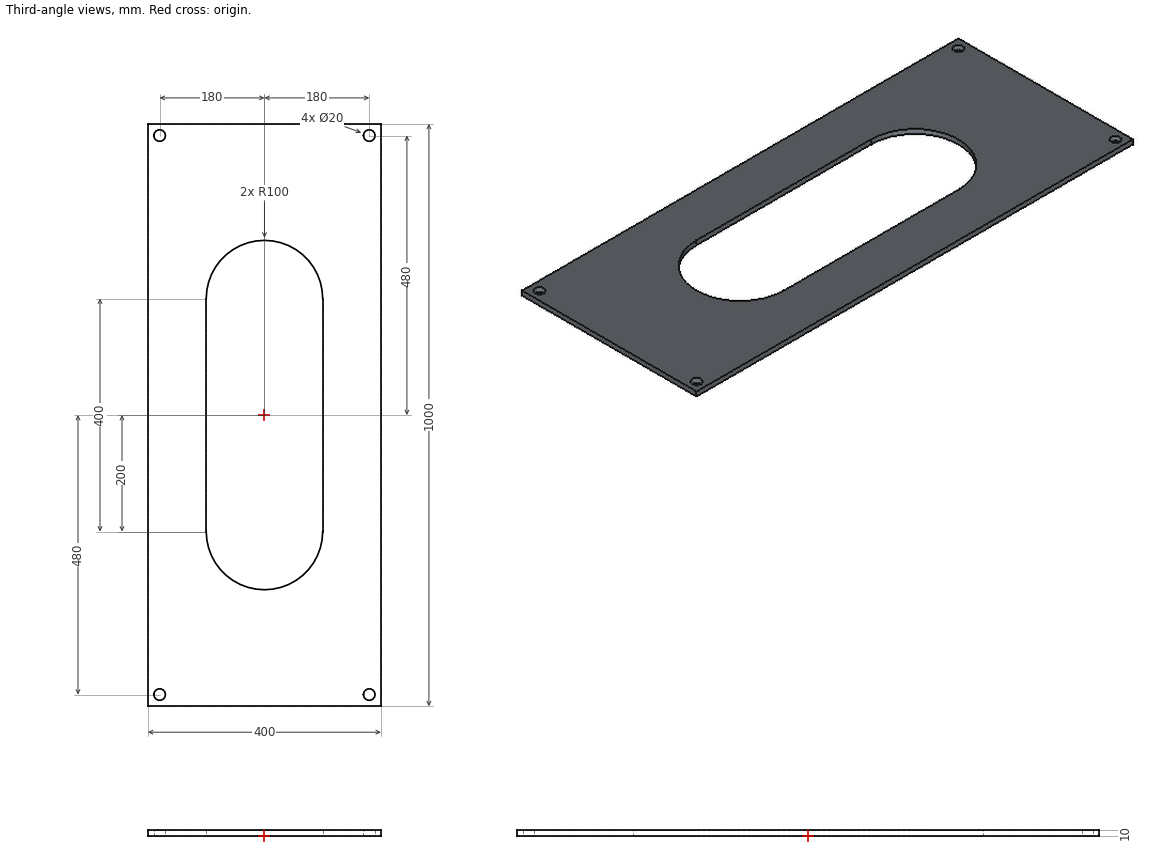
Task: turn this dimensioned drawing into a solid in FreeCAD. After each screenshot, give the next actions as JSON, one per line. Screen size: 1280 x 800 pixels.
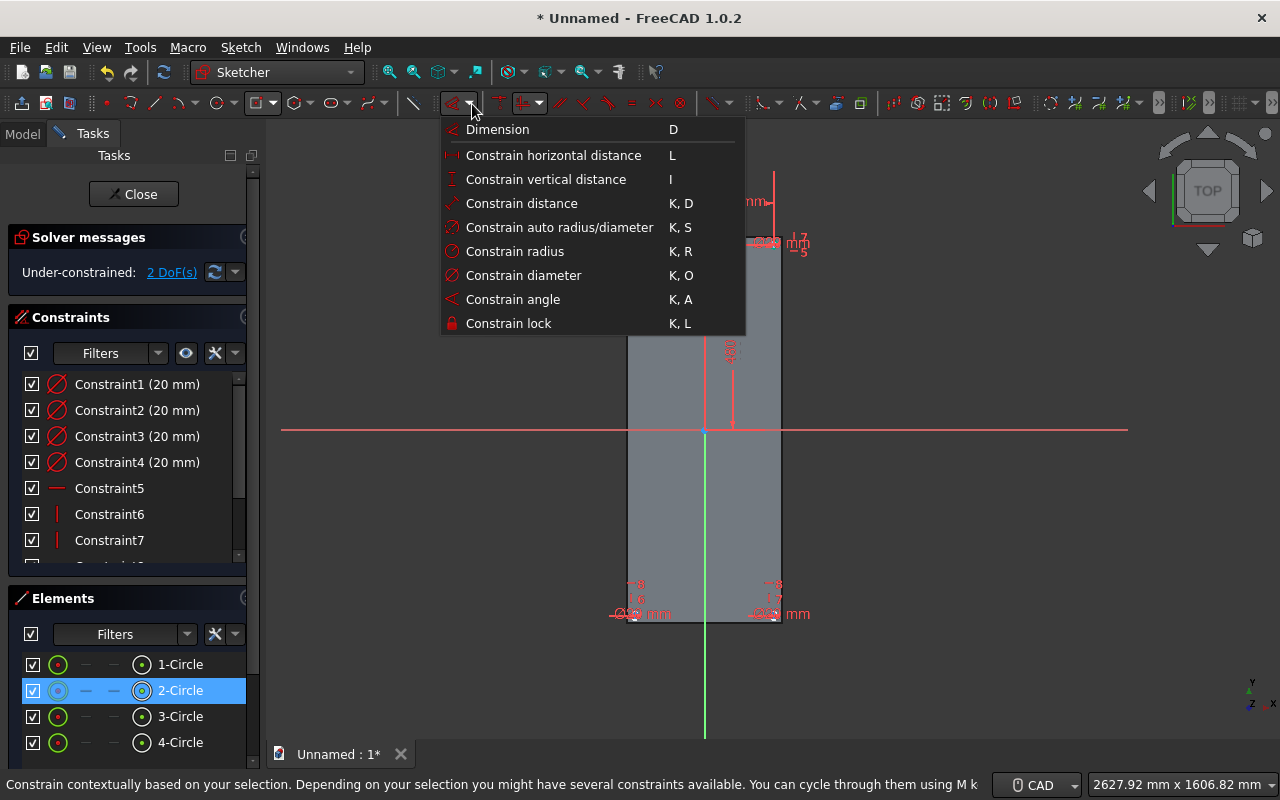
{"action": "left_click", "coordinate": [593, 155]}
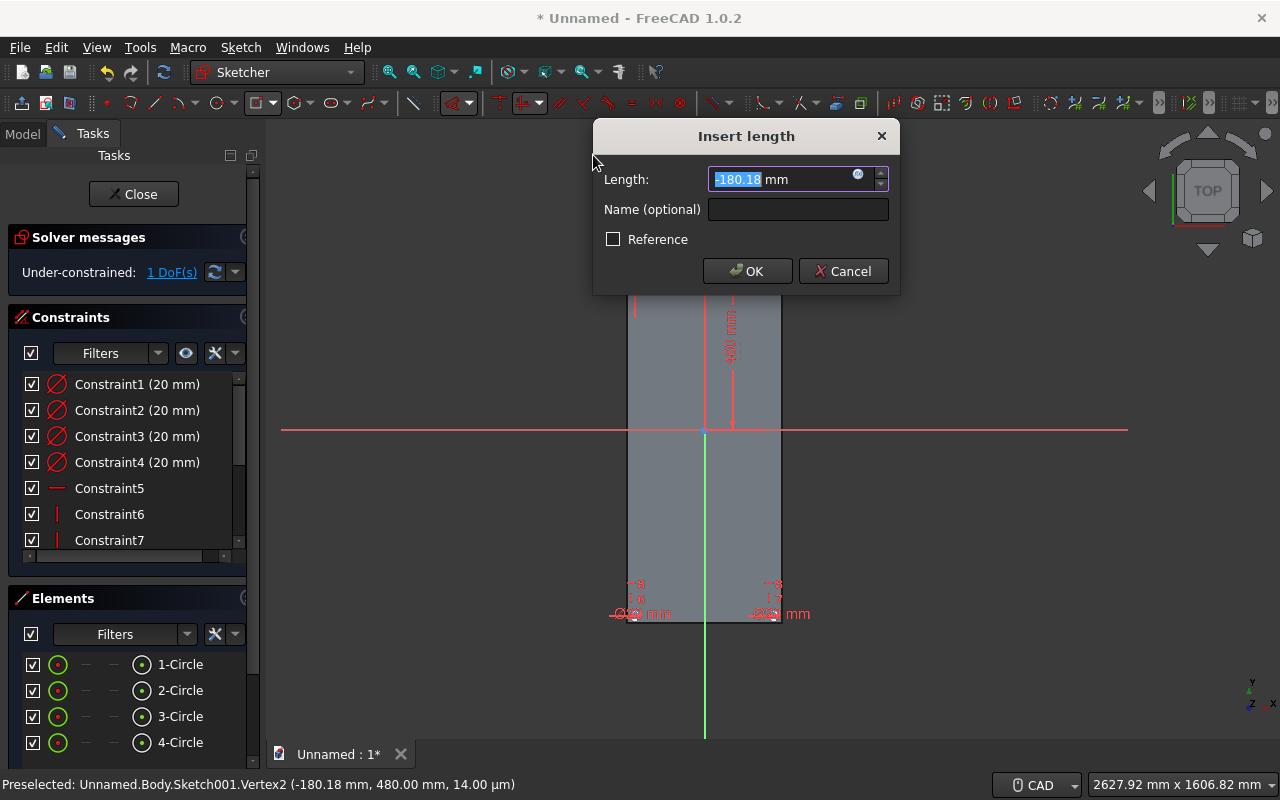
{"action": "type", "text": "-180"}
{"action": "key", "text": "Return"}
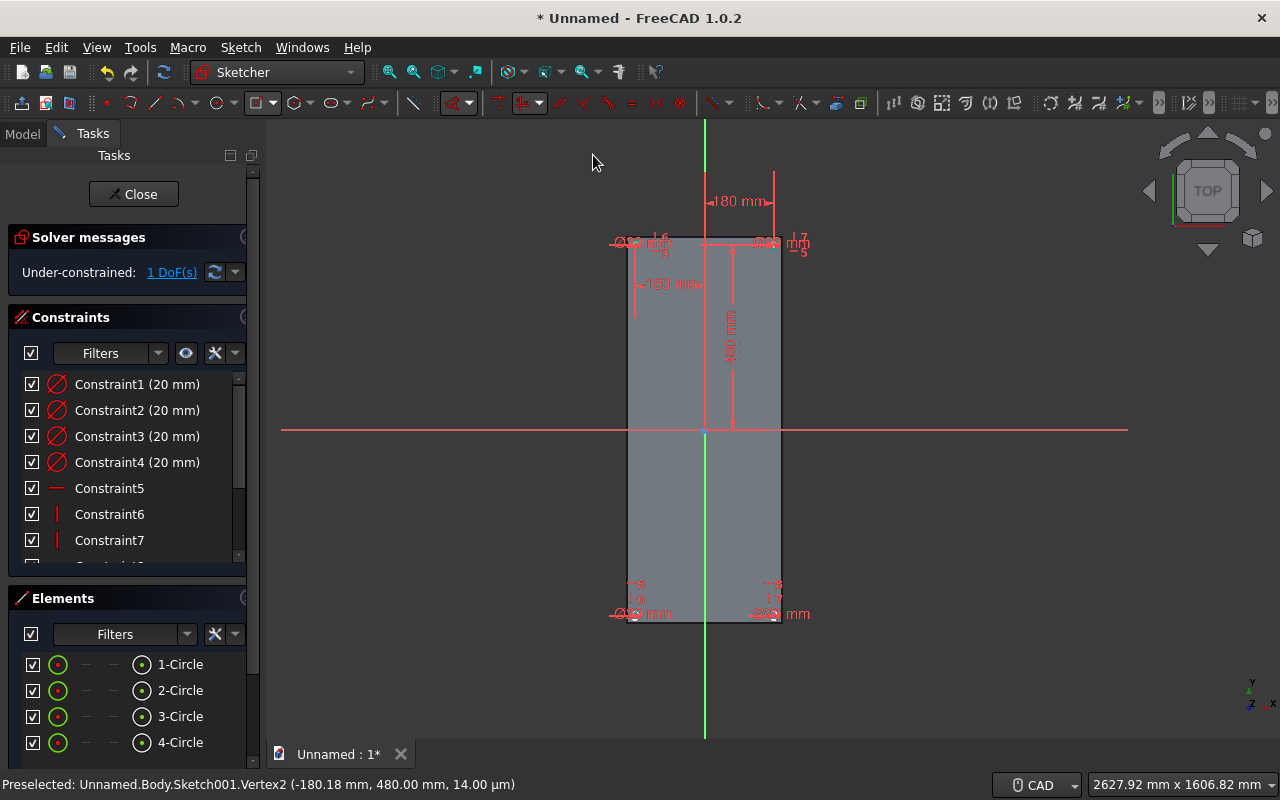
{"action": "left_click", "coordinate": [635, 616]}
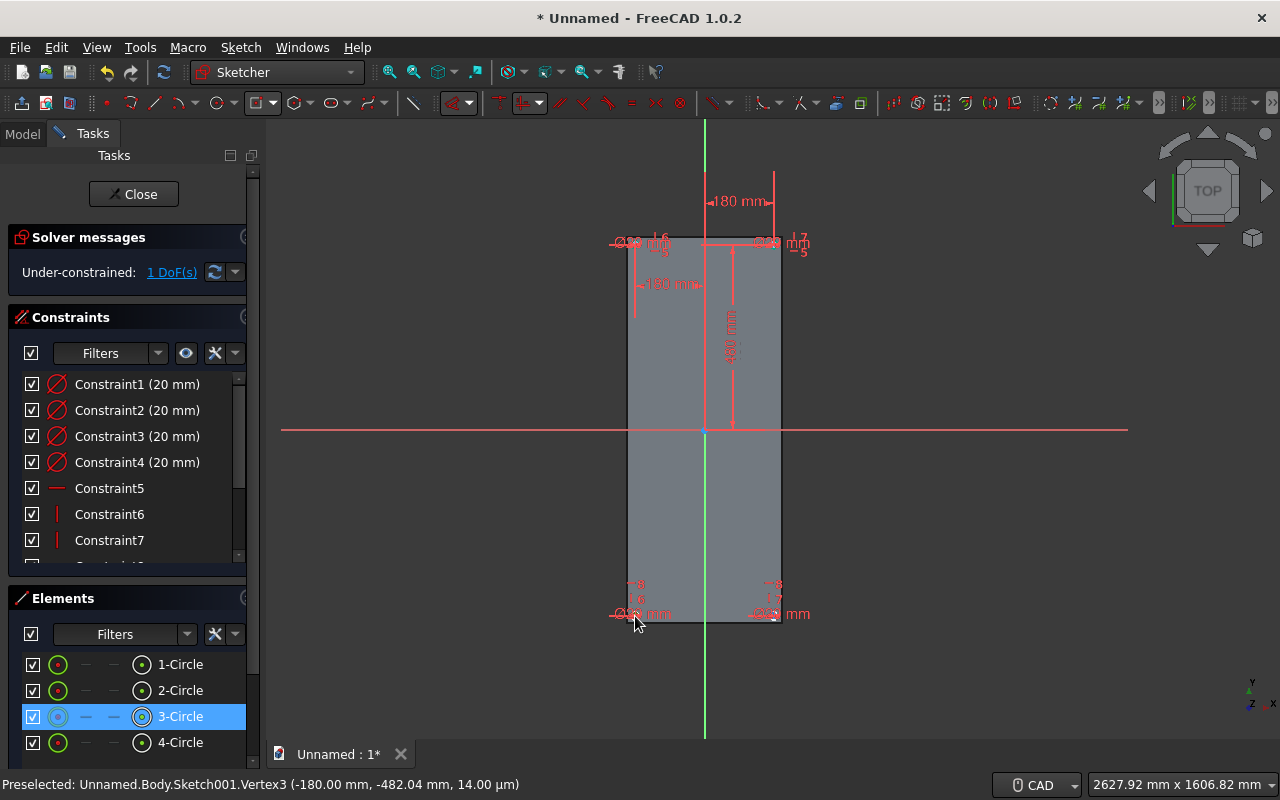
{"action": "left_click", "coordinate": [472, 104]}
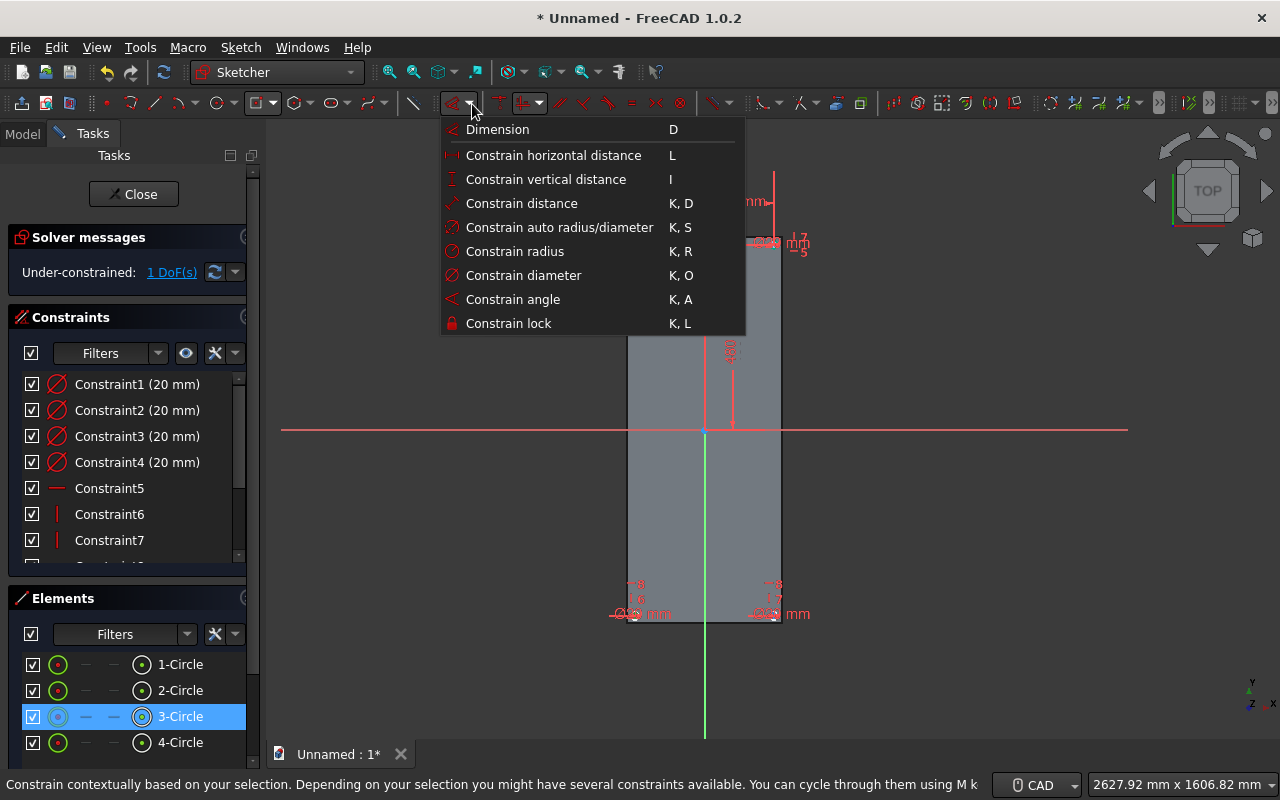
{"action": "left_click", "coordinate": [593, 179]}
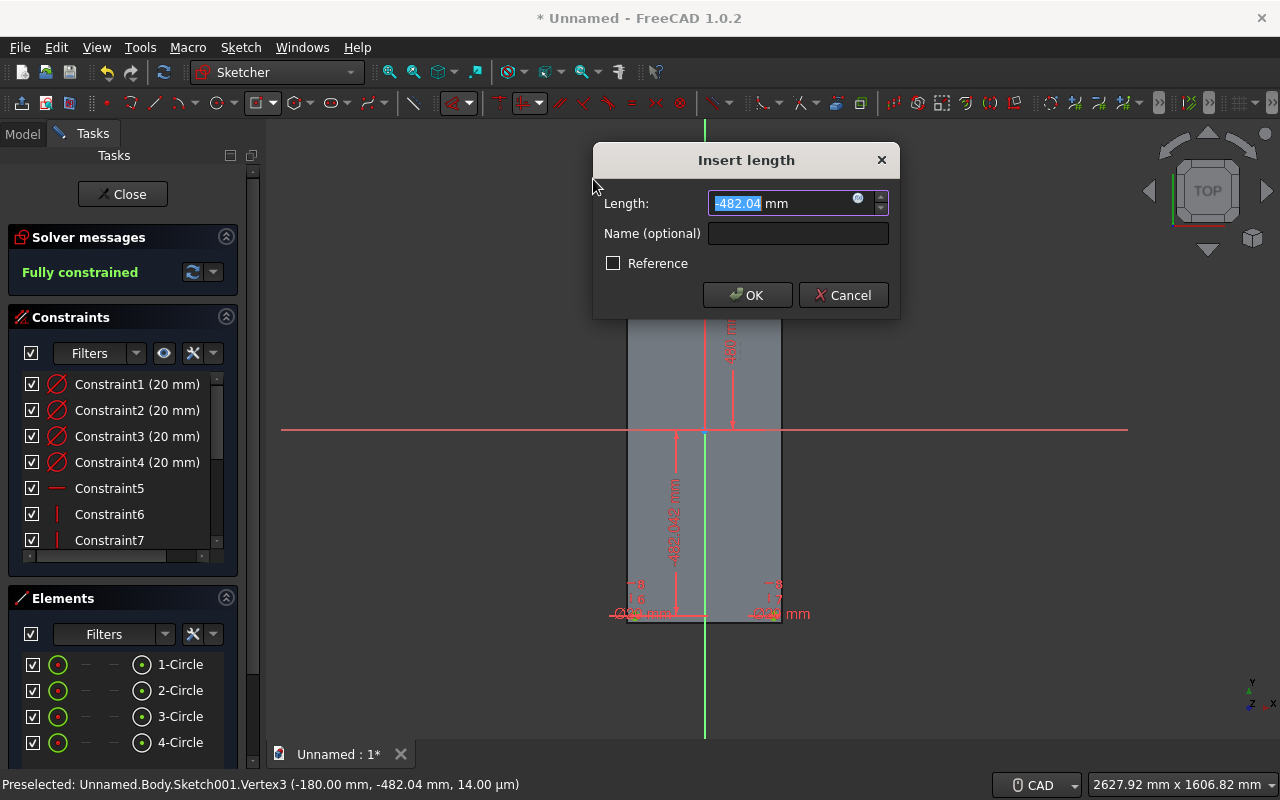
{"action": "type", "text": "-480"}
{"action": "key", "text": "Return"}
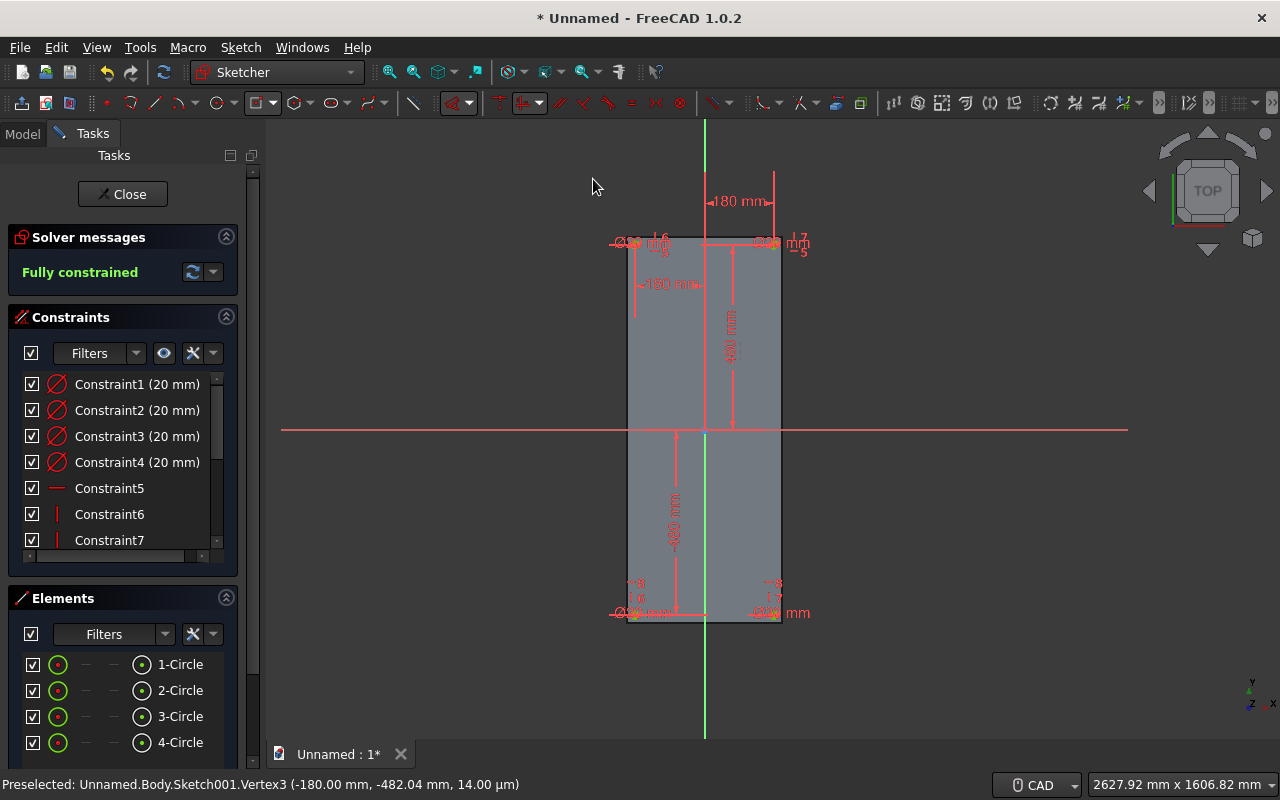
{"action": "left_click", "coordinate": [123, 194]}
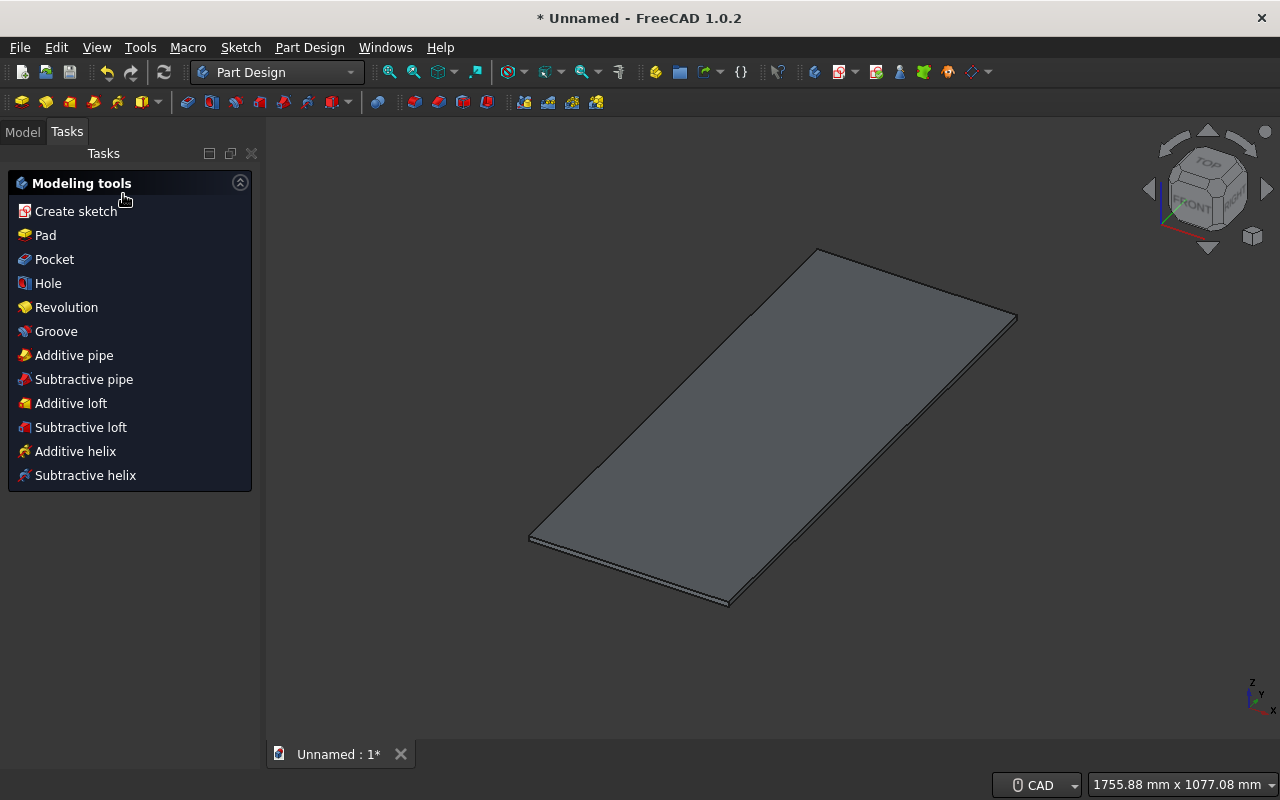
{"action": "left_click", "coordinate": [188, 102]}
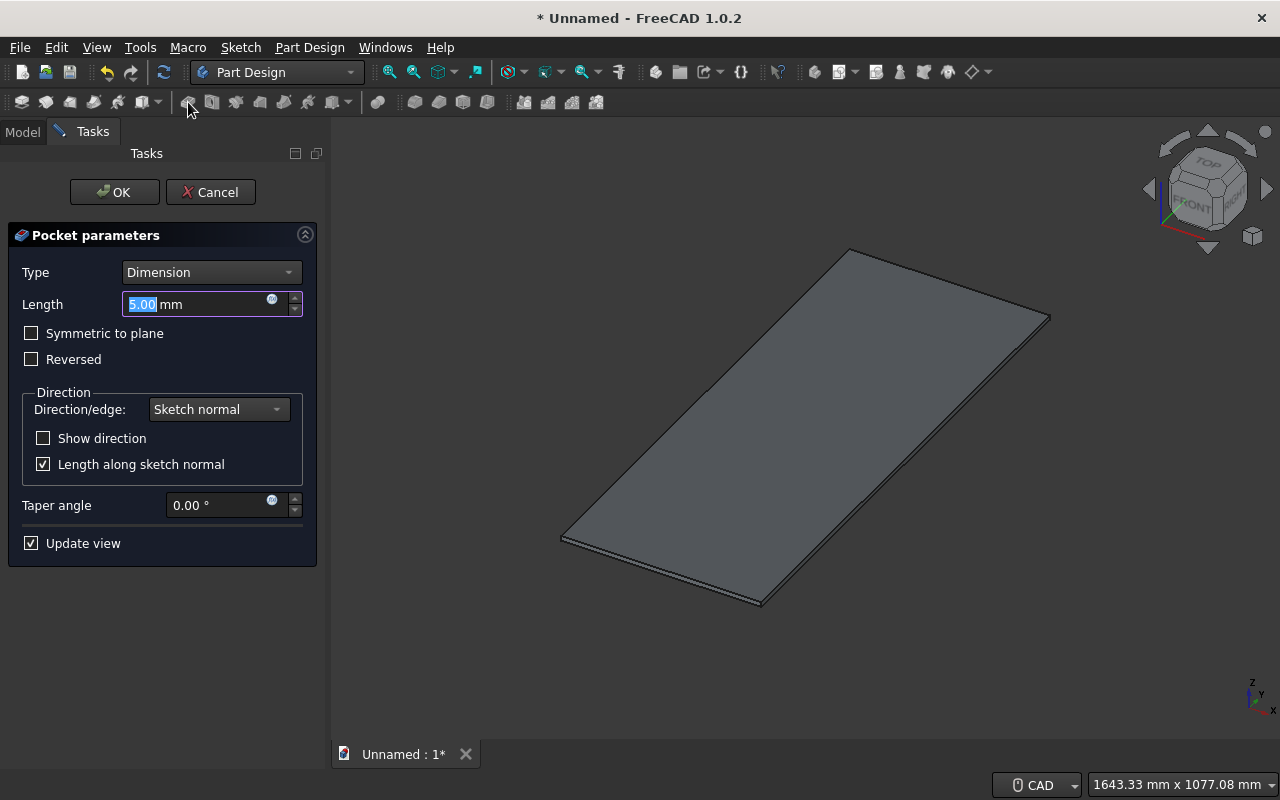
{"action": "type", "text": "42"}
{"action": "key", "text": "Tab"}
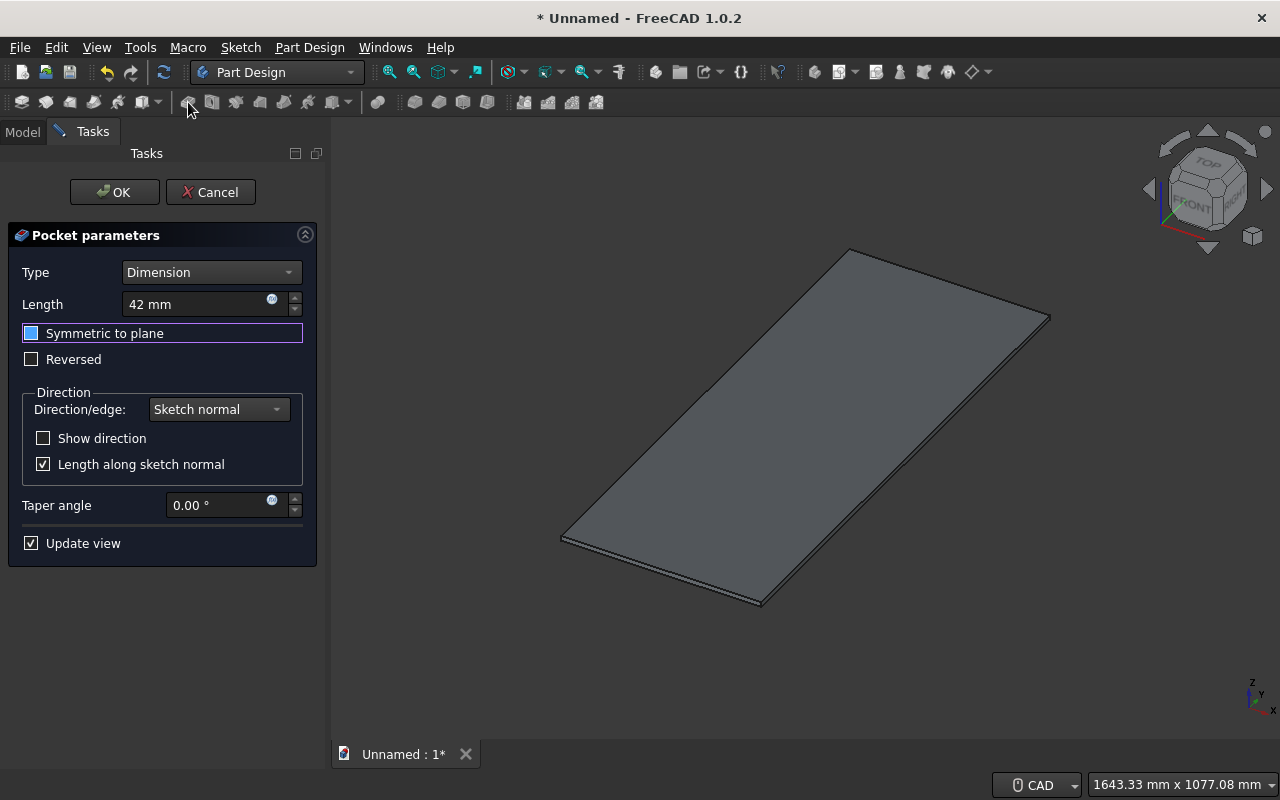
{"action": "left_click", "coordinate": [30, 359]}